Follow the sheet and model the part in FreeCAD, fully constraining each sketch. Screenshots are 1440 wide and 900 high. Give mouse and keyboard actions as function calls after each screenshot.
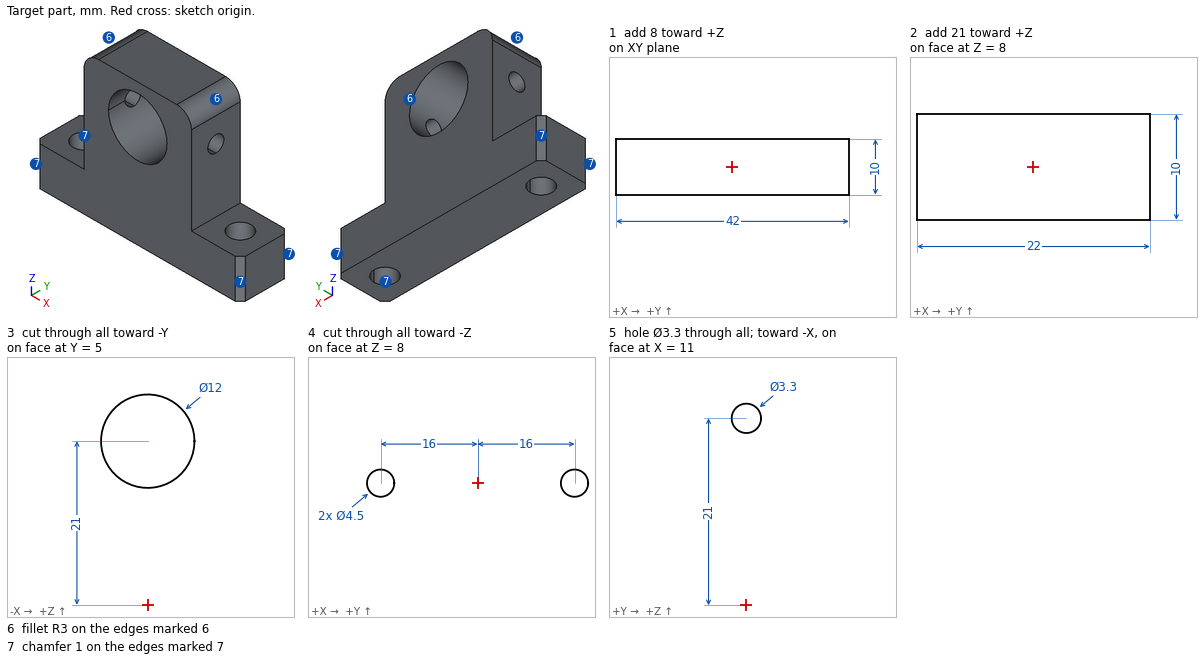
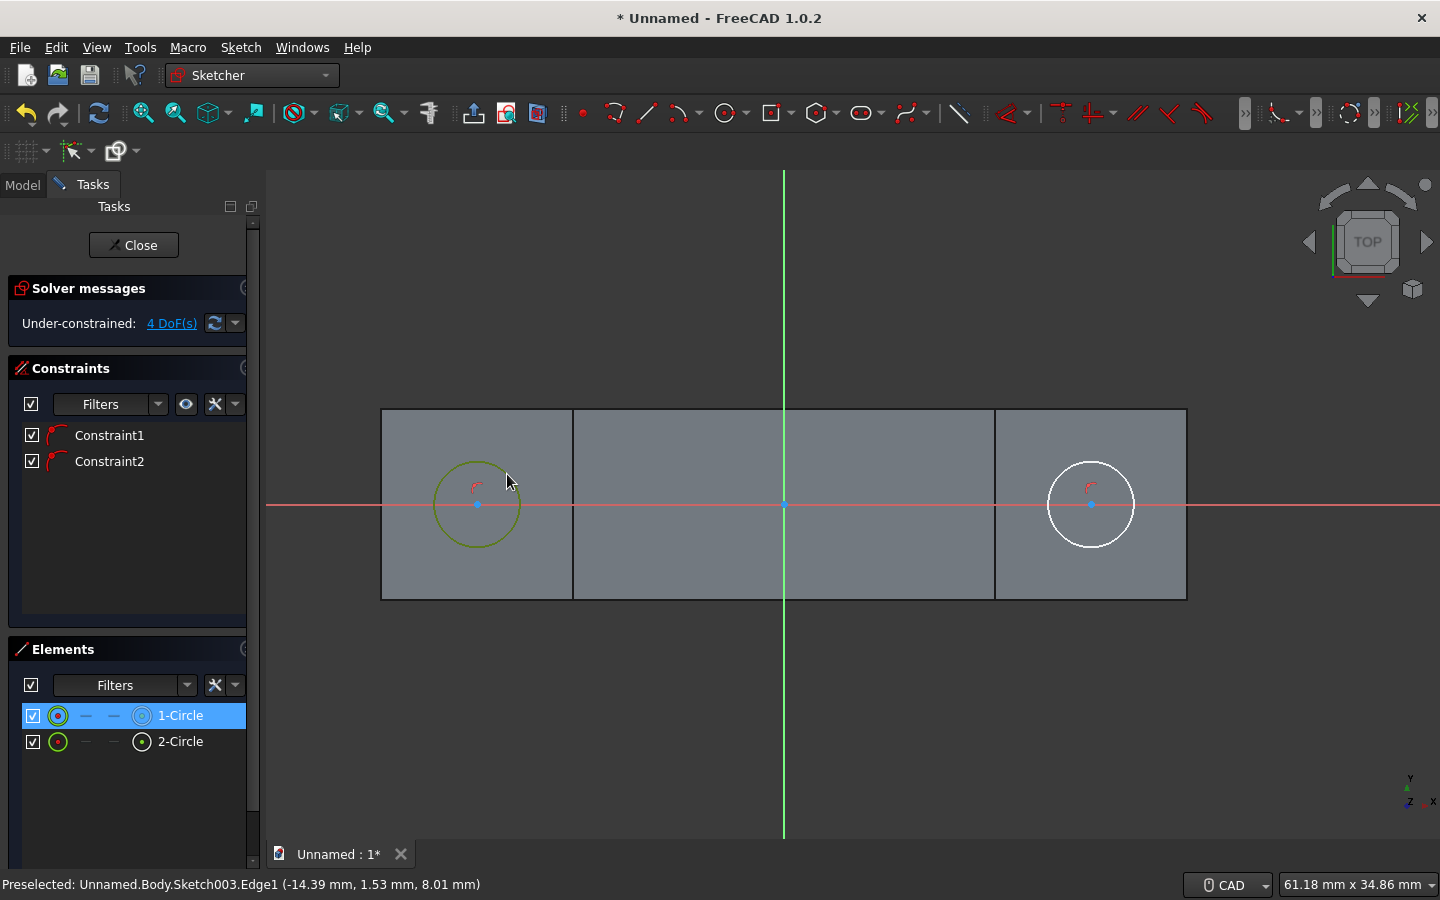
click(1121, 474)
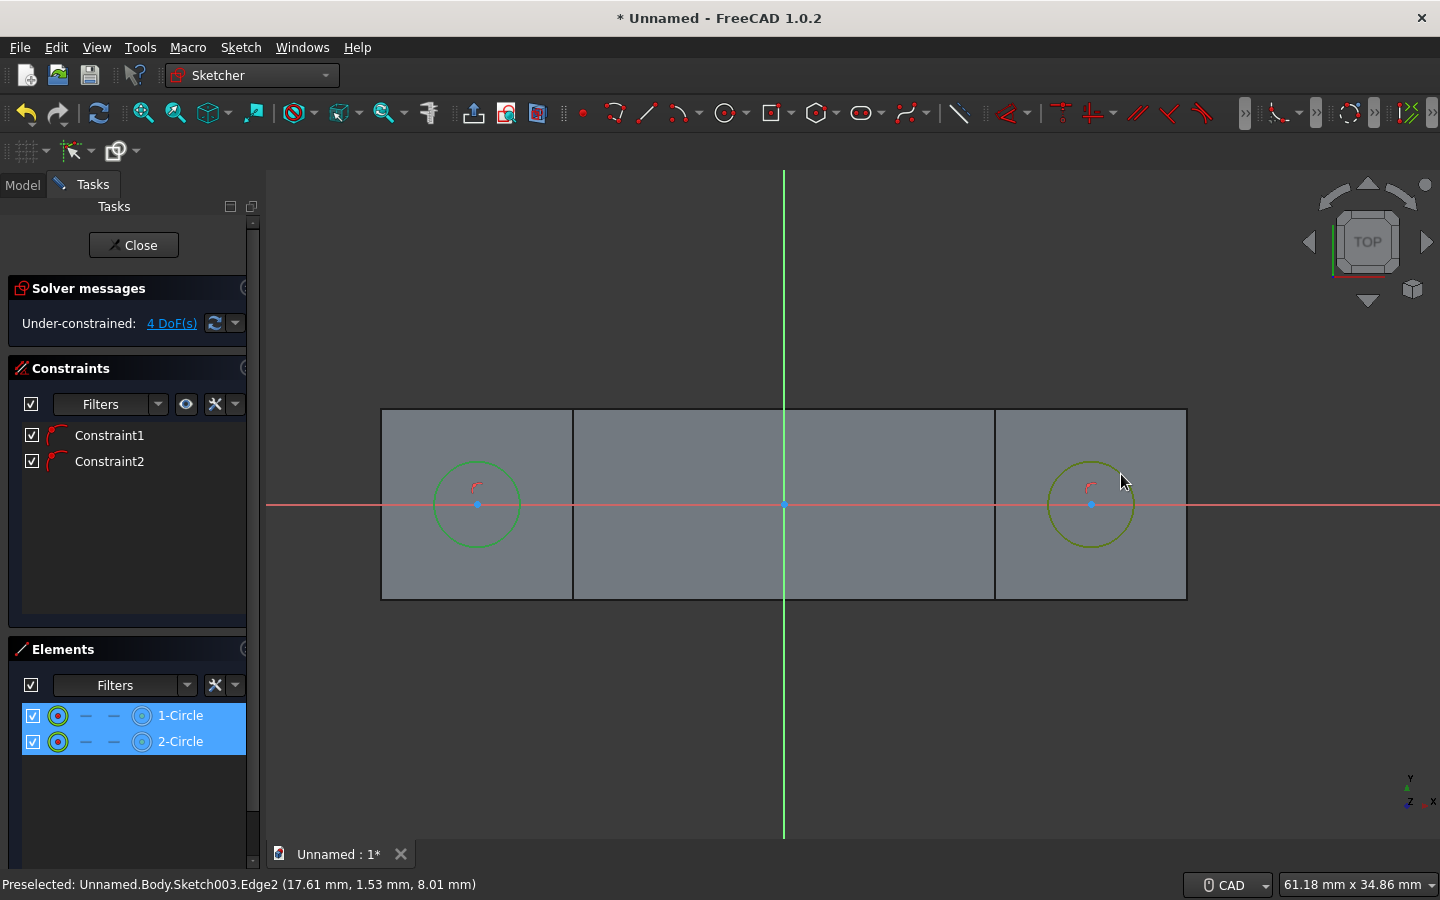
key(e)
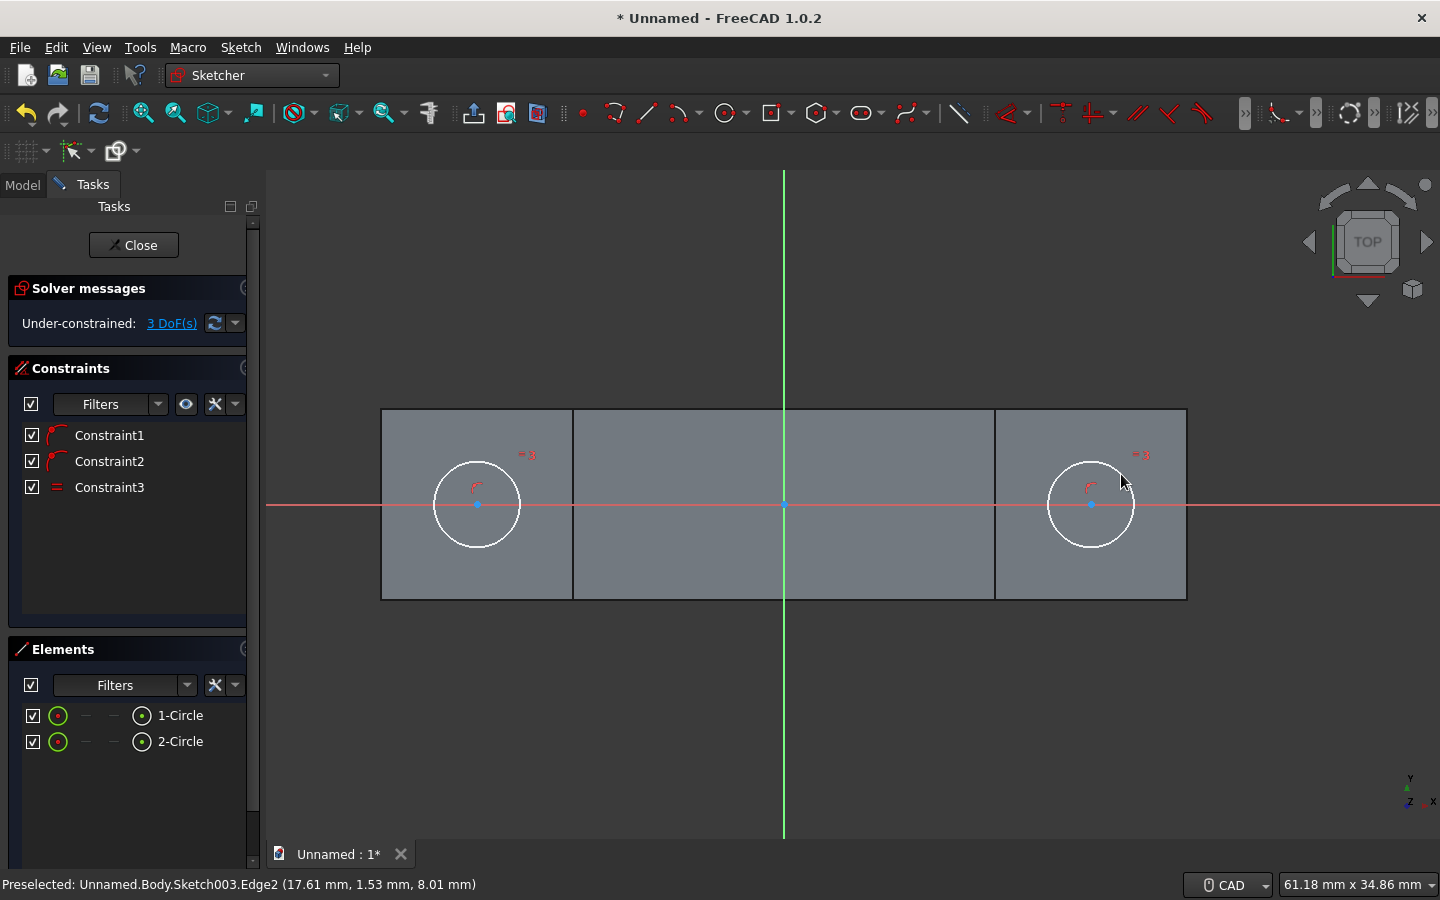
click(1006, 114)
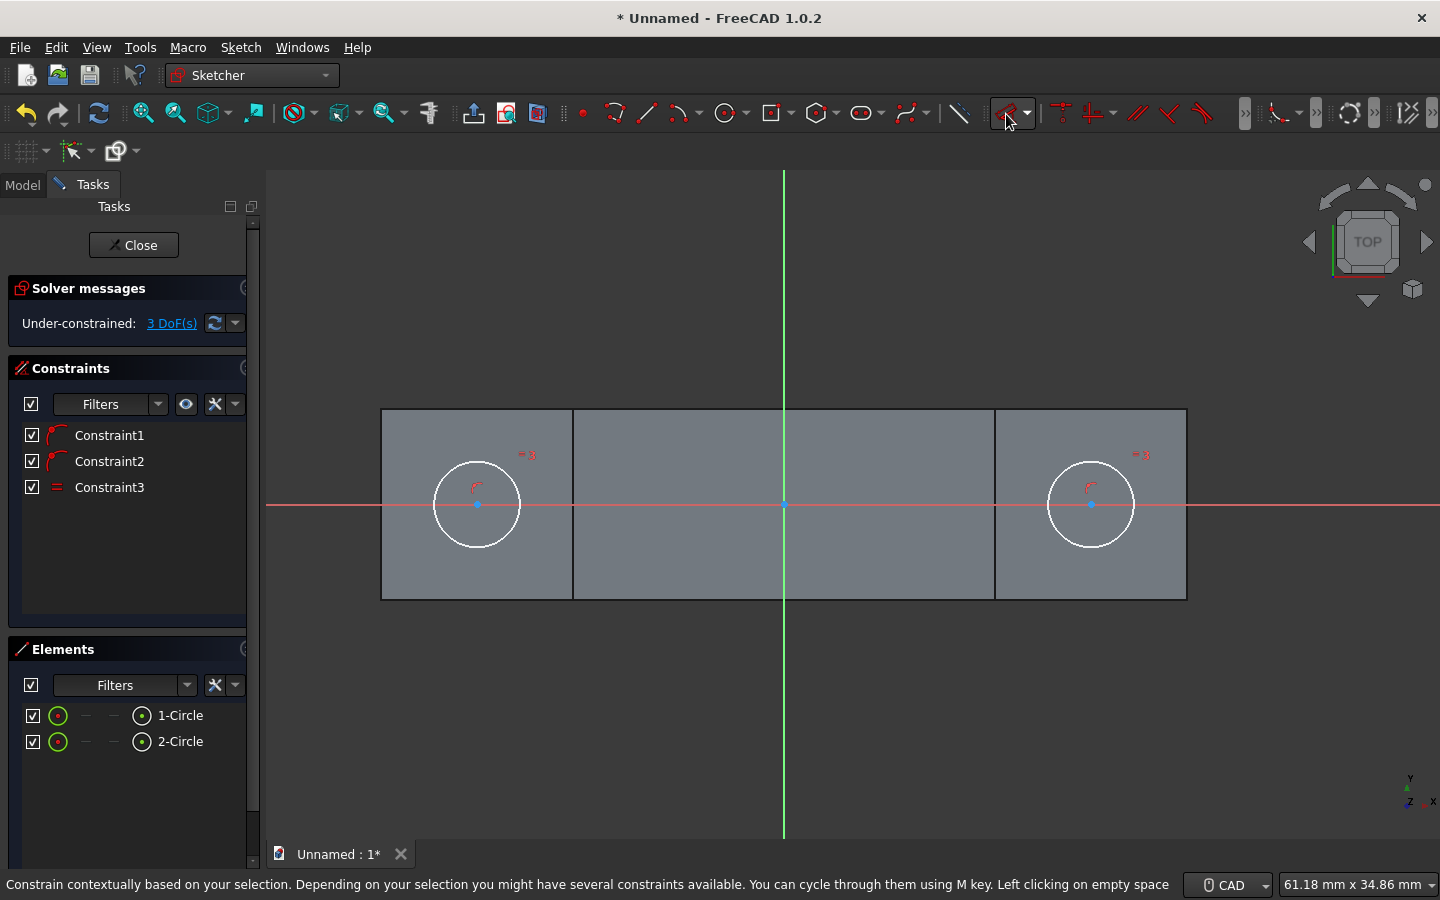
click(507, 474)
click(529, 451)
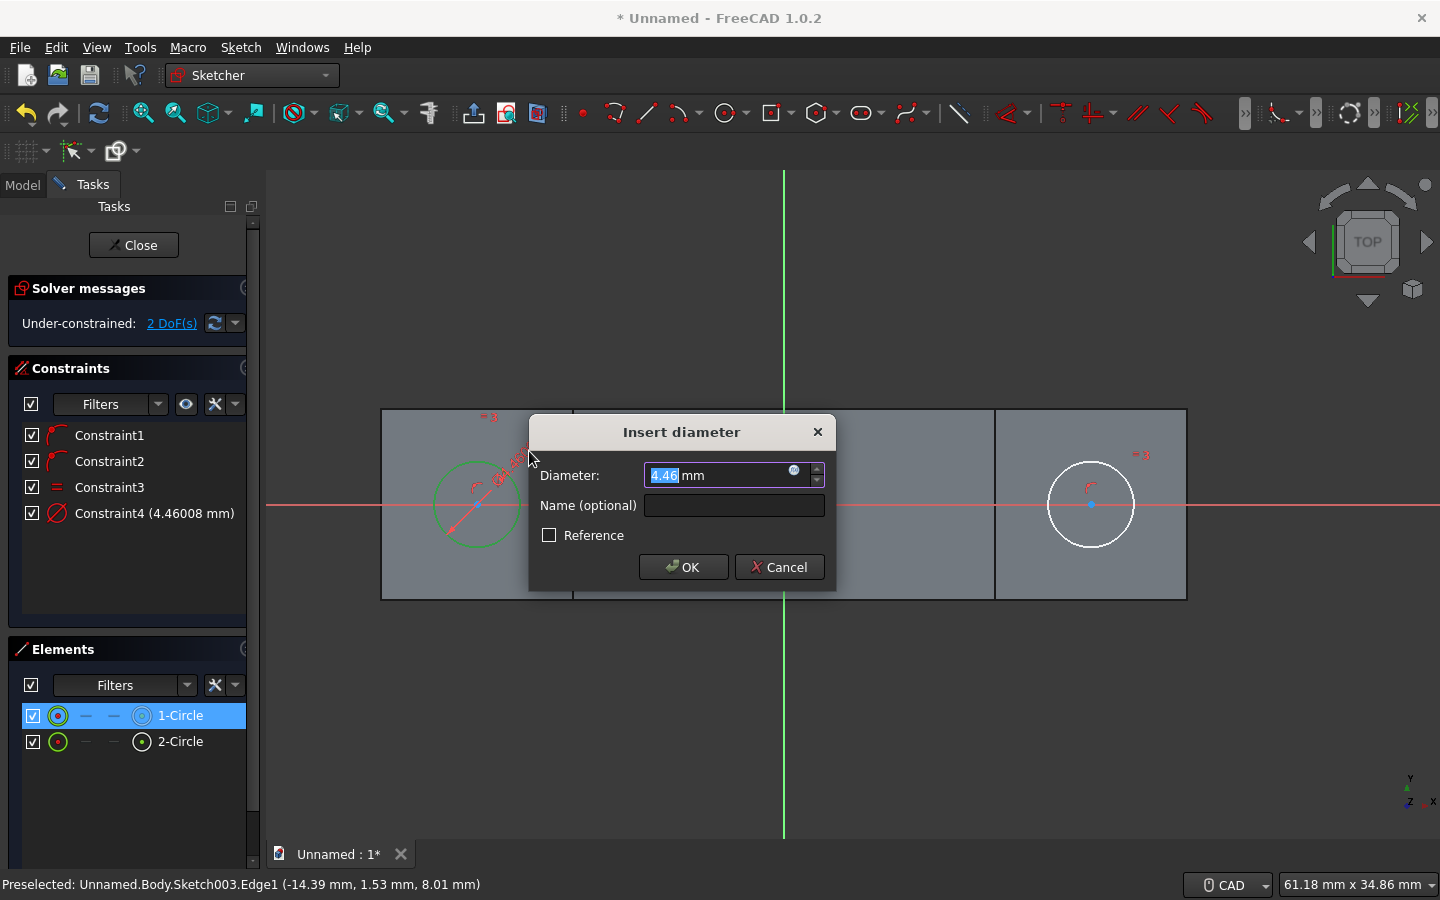
text(4.5)
key(Return)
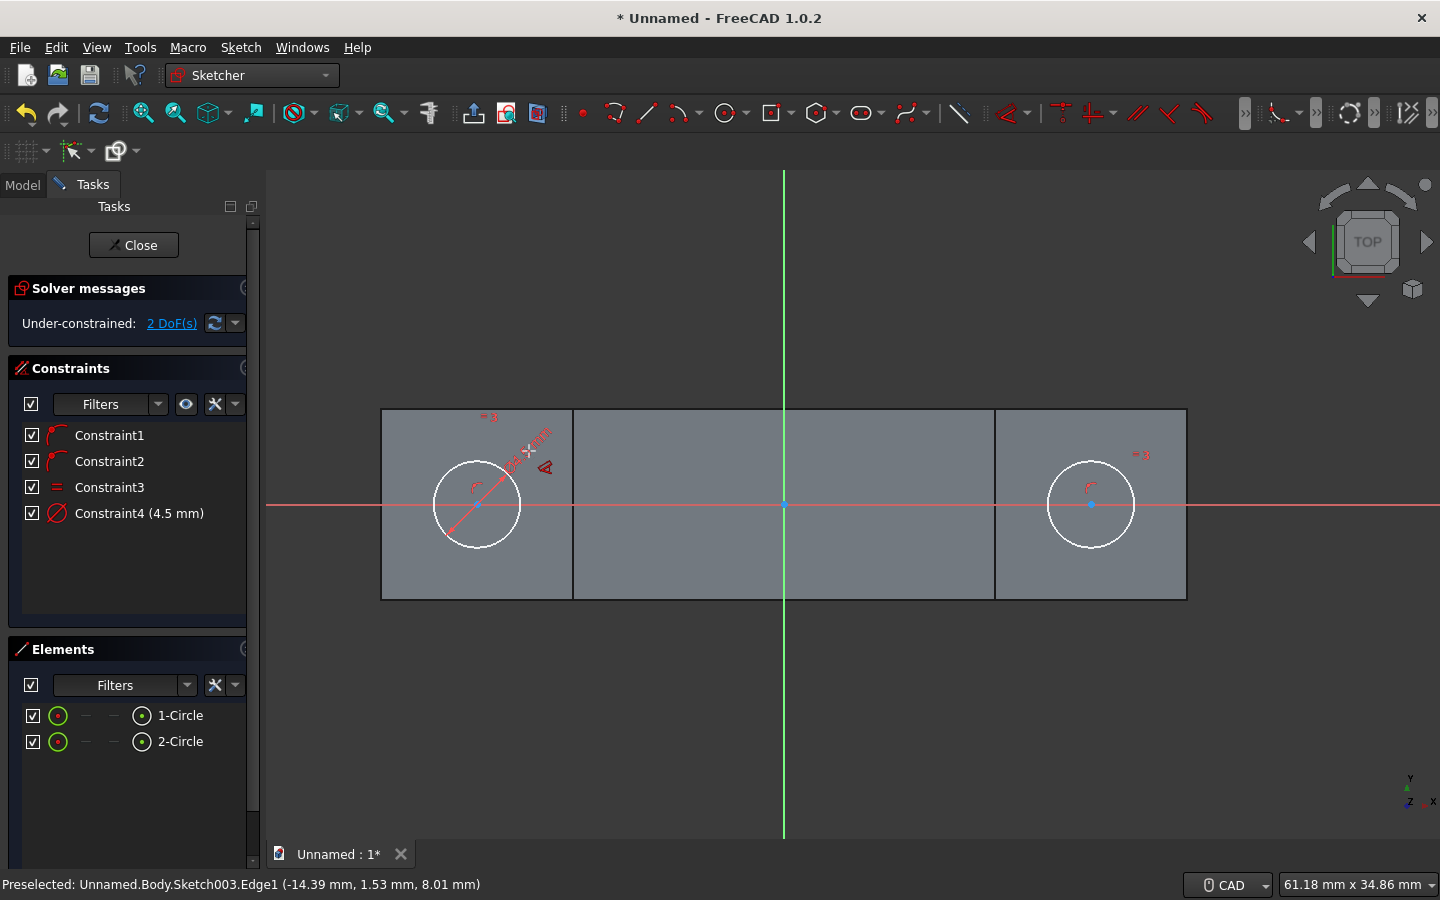
click(477, 504)
click(631, 538)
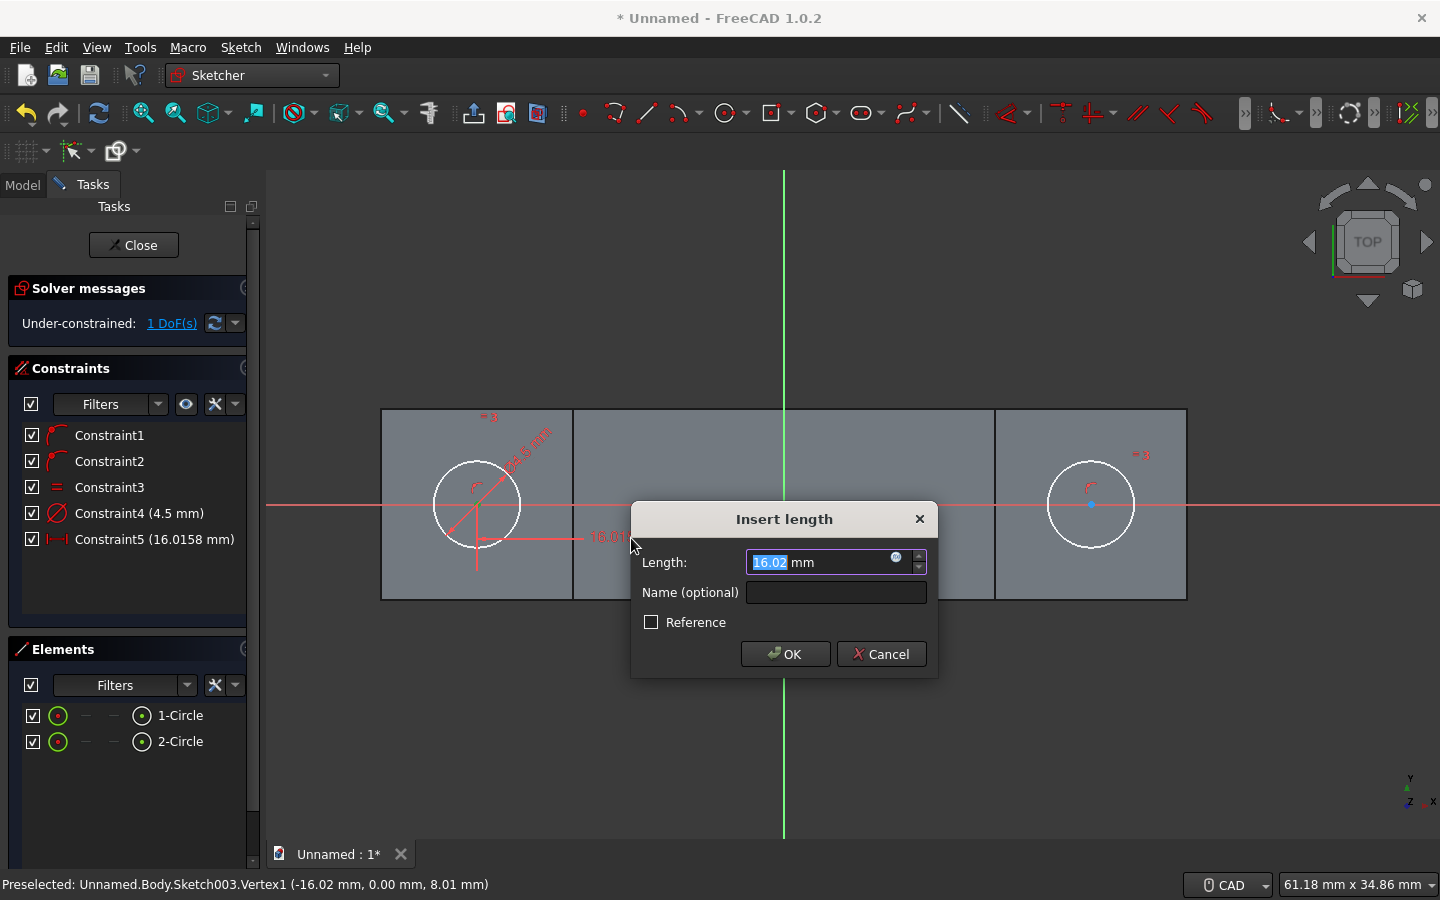
text(16)
key(Return)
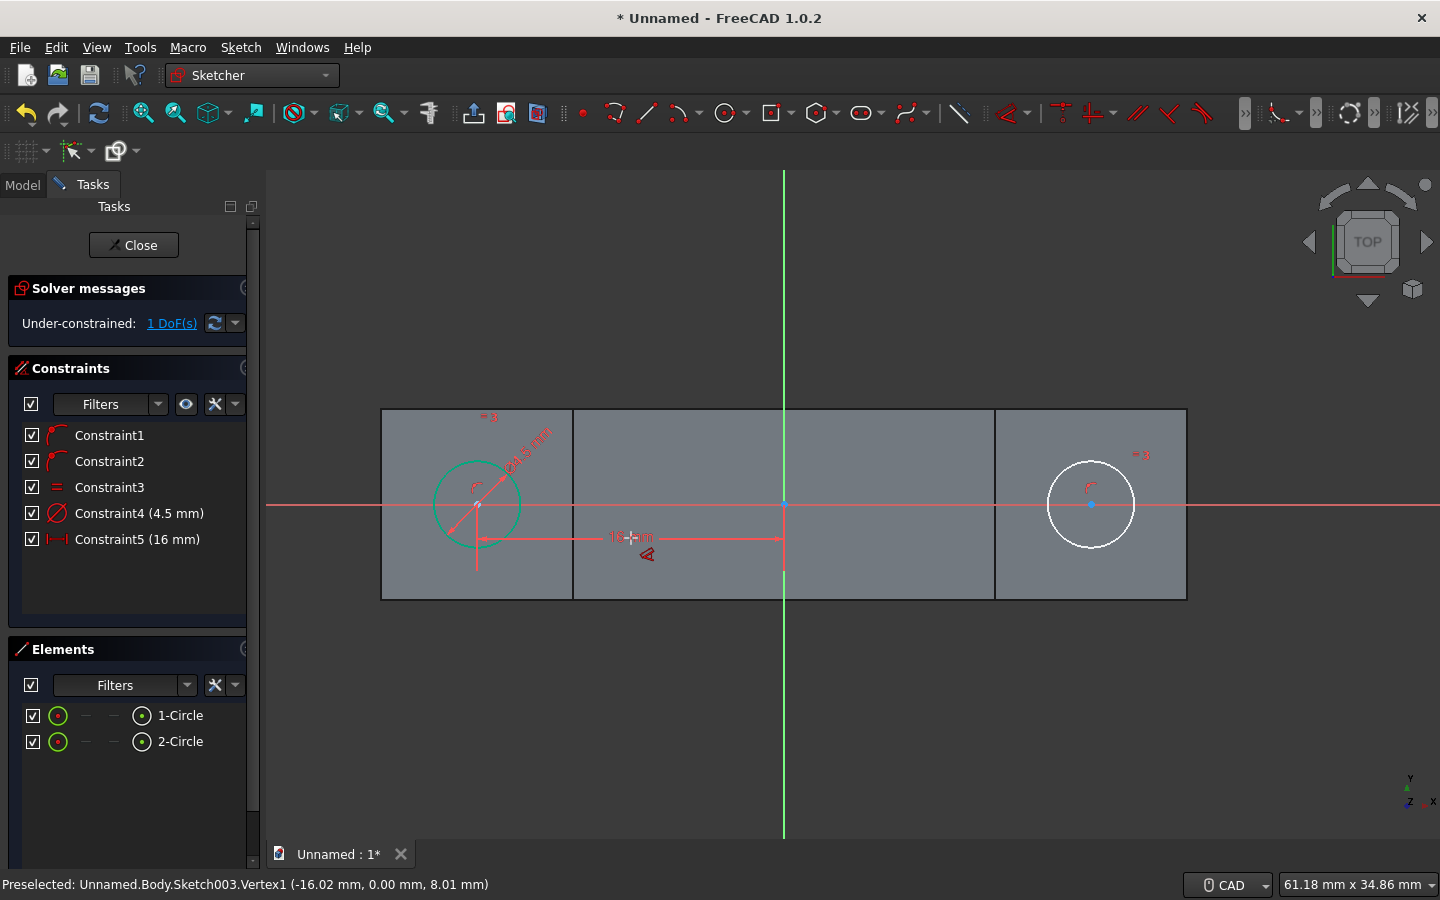
click(1091, 504)
click(938, 538)